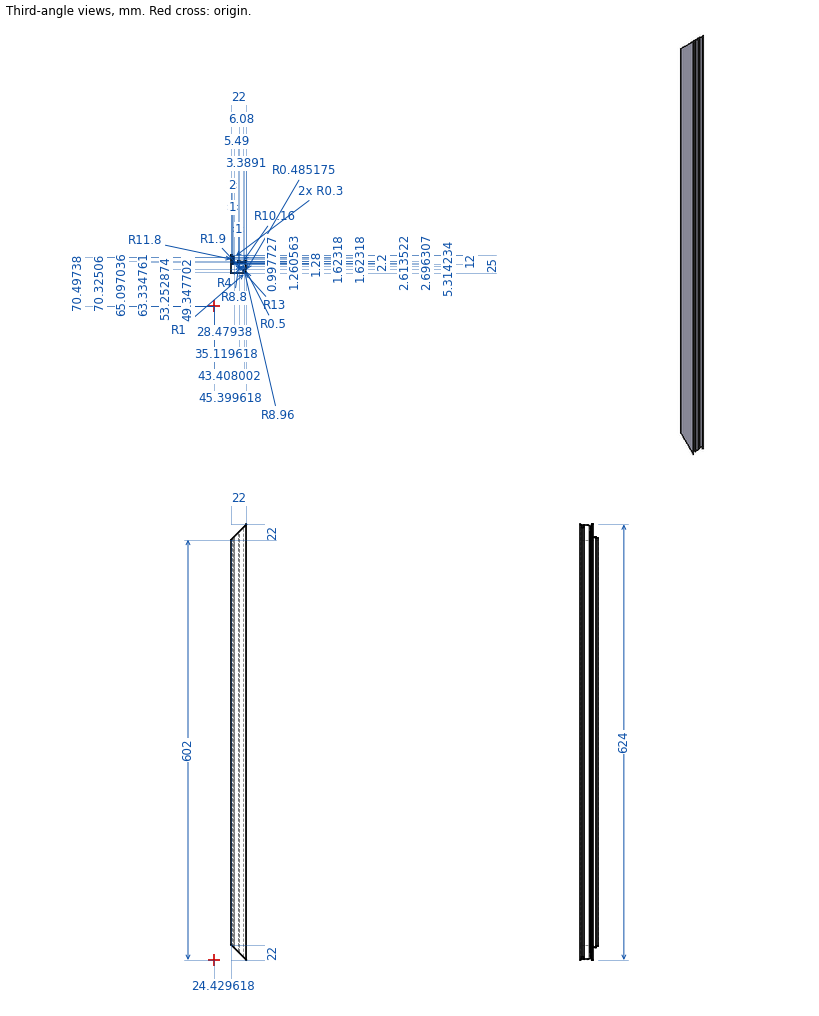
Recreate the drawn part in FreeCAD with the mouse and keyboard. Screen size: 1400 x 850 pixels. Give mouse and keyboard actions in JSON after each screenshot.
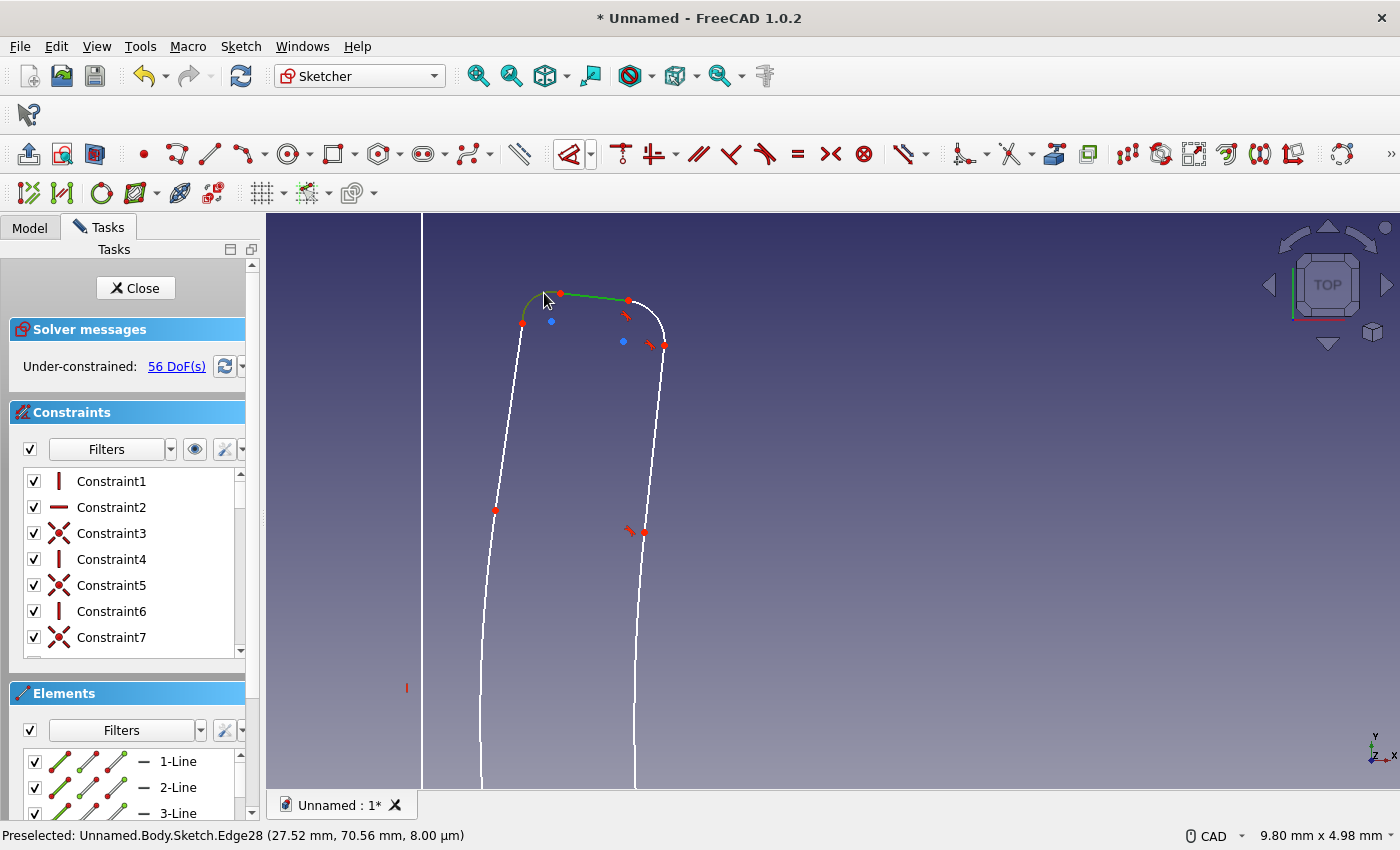
{"action": "key", "text": "t"}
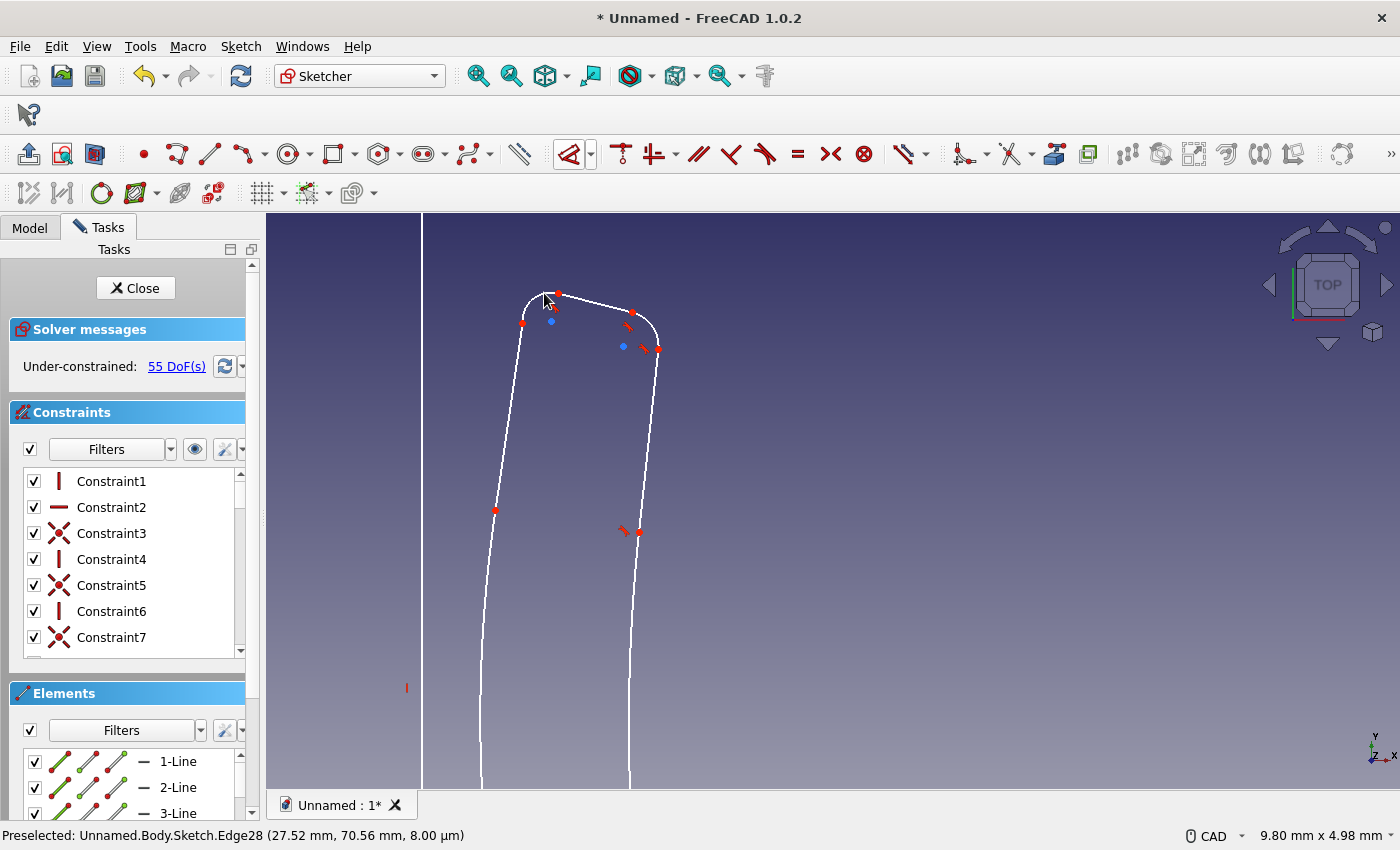
{"action": "scroll", "coordinate": [655, 355], "scroll_direction": "down", "scroll_amount": 10}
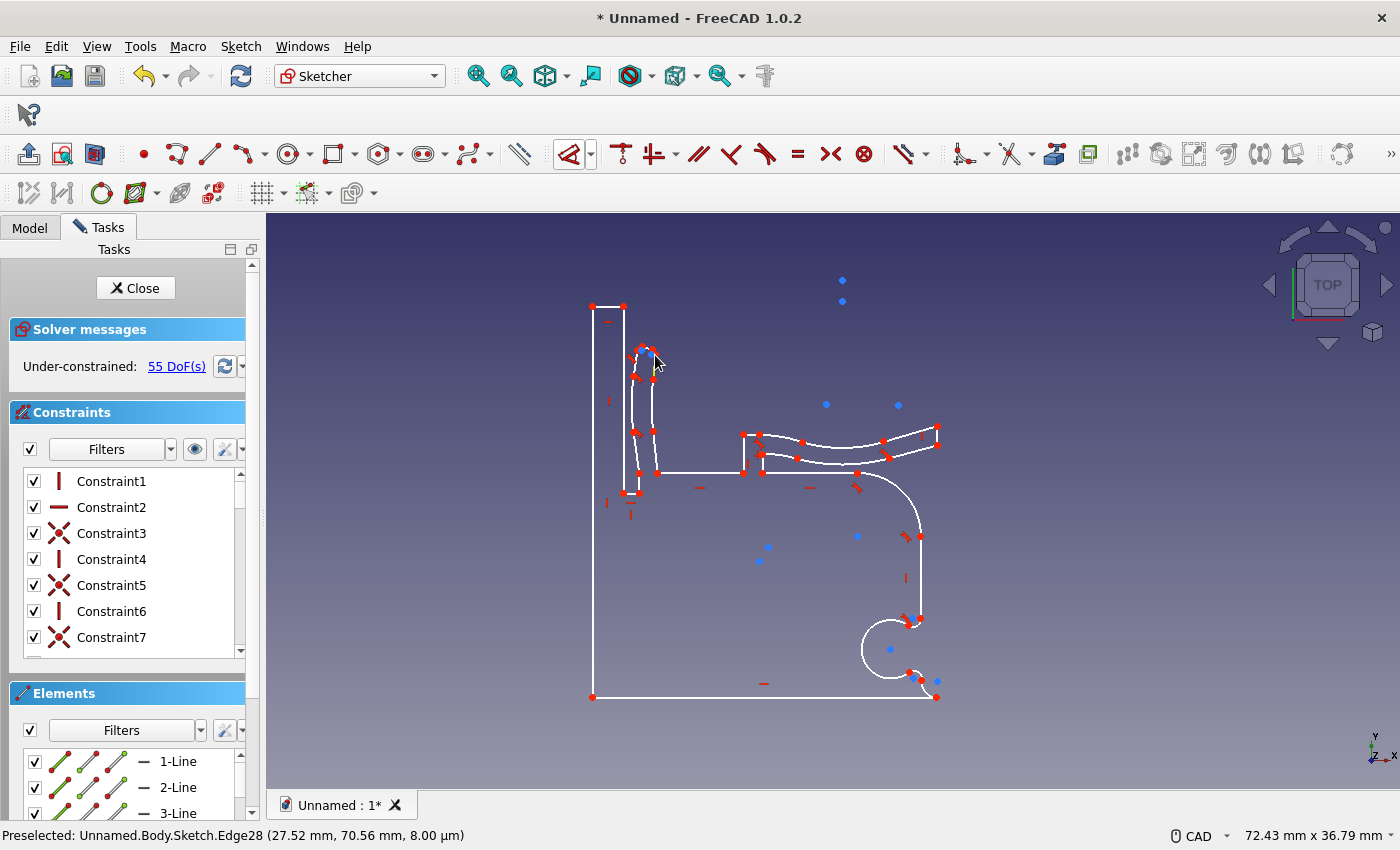
{"action": "scroll", "coordinate": [636, 359], "scroll_direction": "up", "scroll_amount": 3}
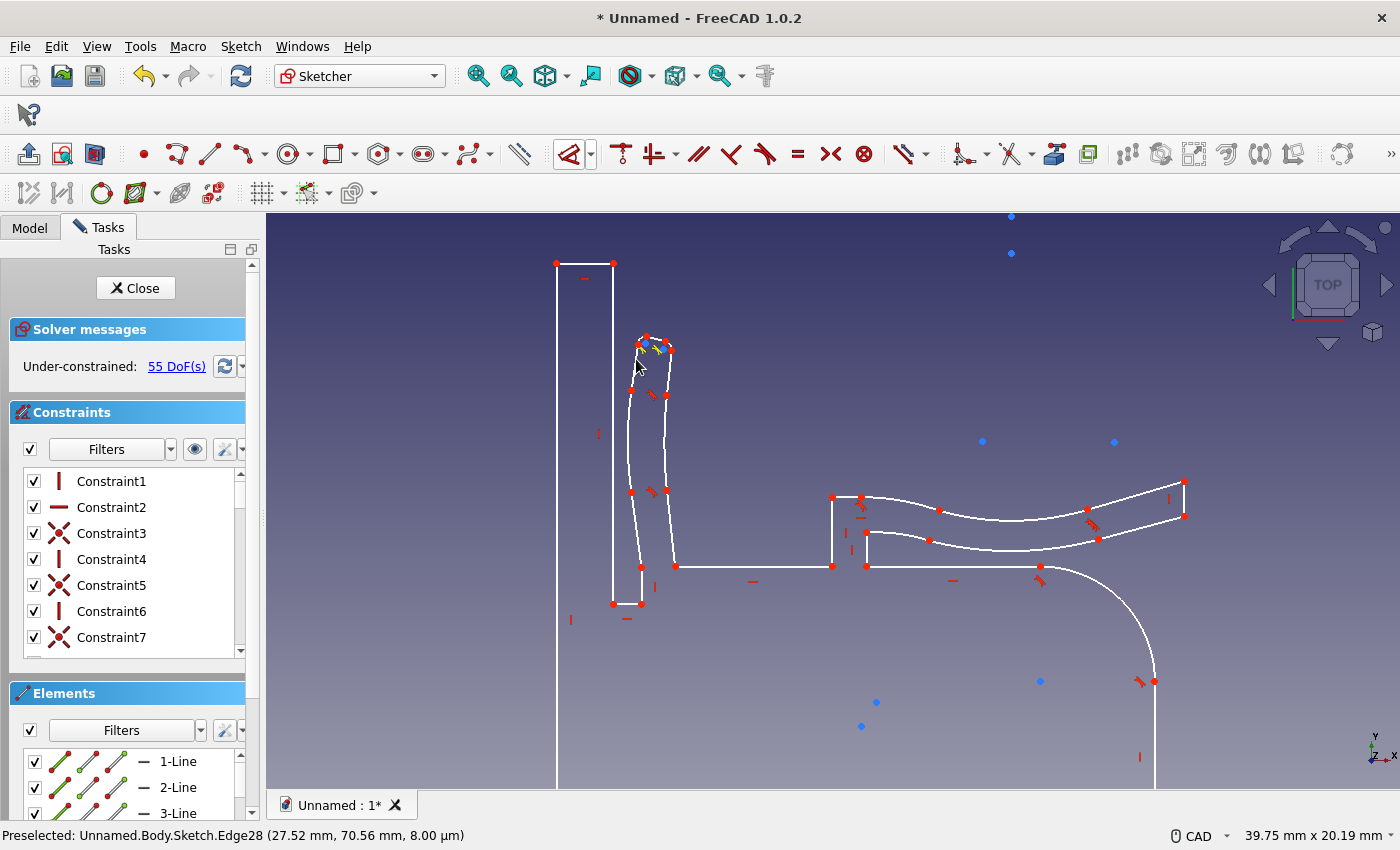
{"action": "left_click", "coordinate": [636, 358]}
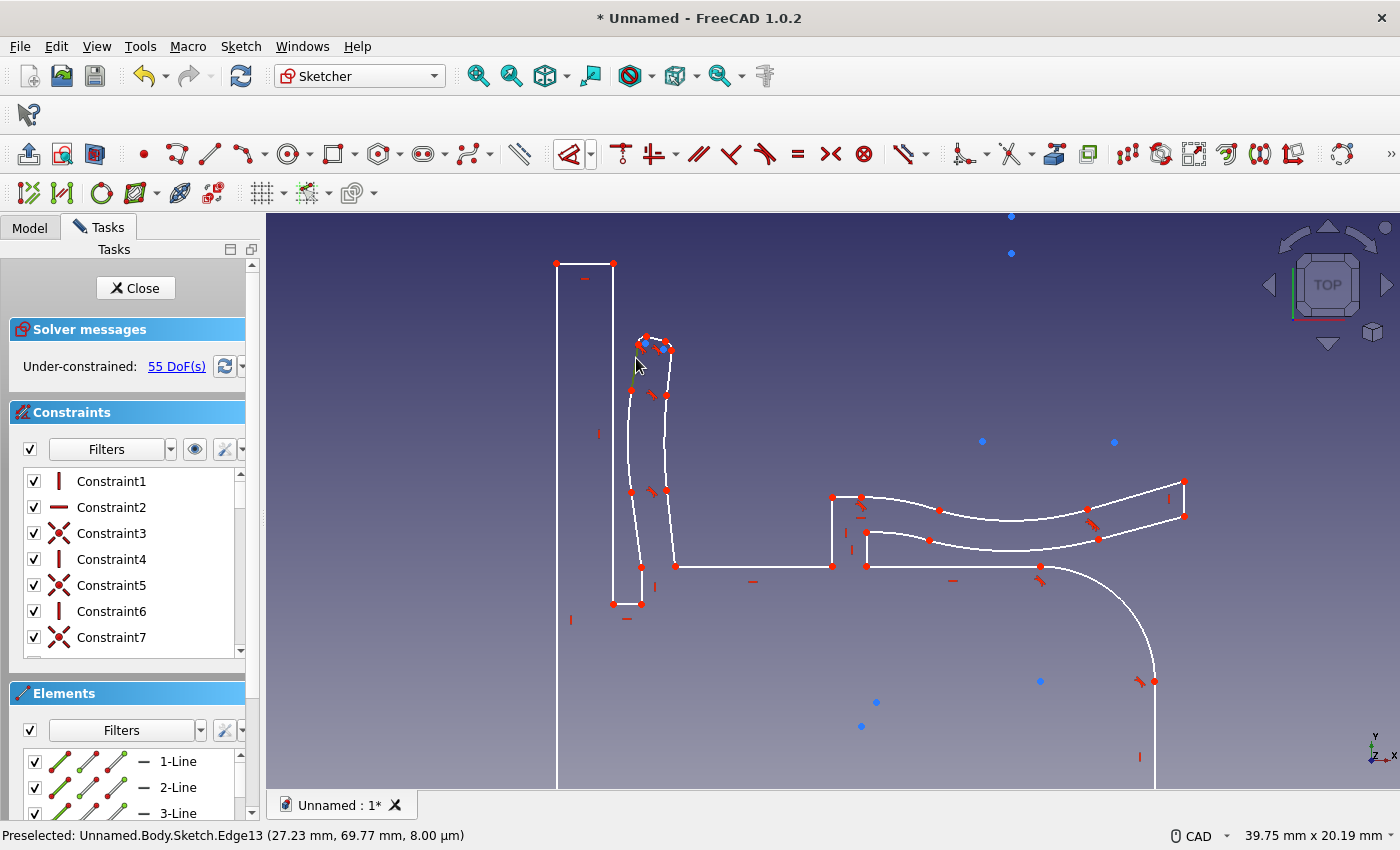
{"action": "scroll", "coordinate": [641, 338], "scroll_direction": "up", "scroll_amount": 4}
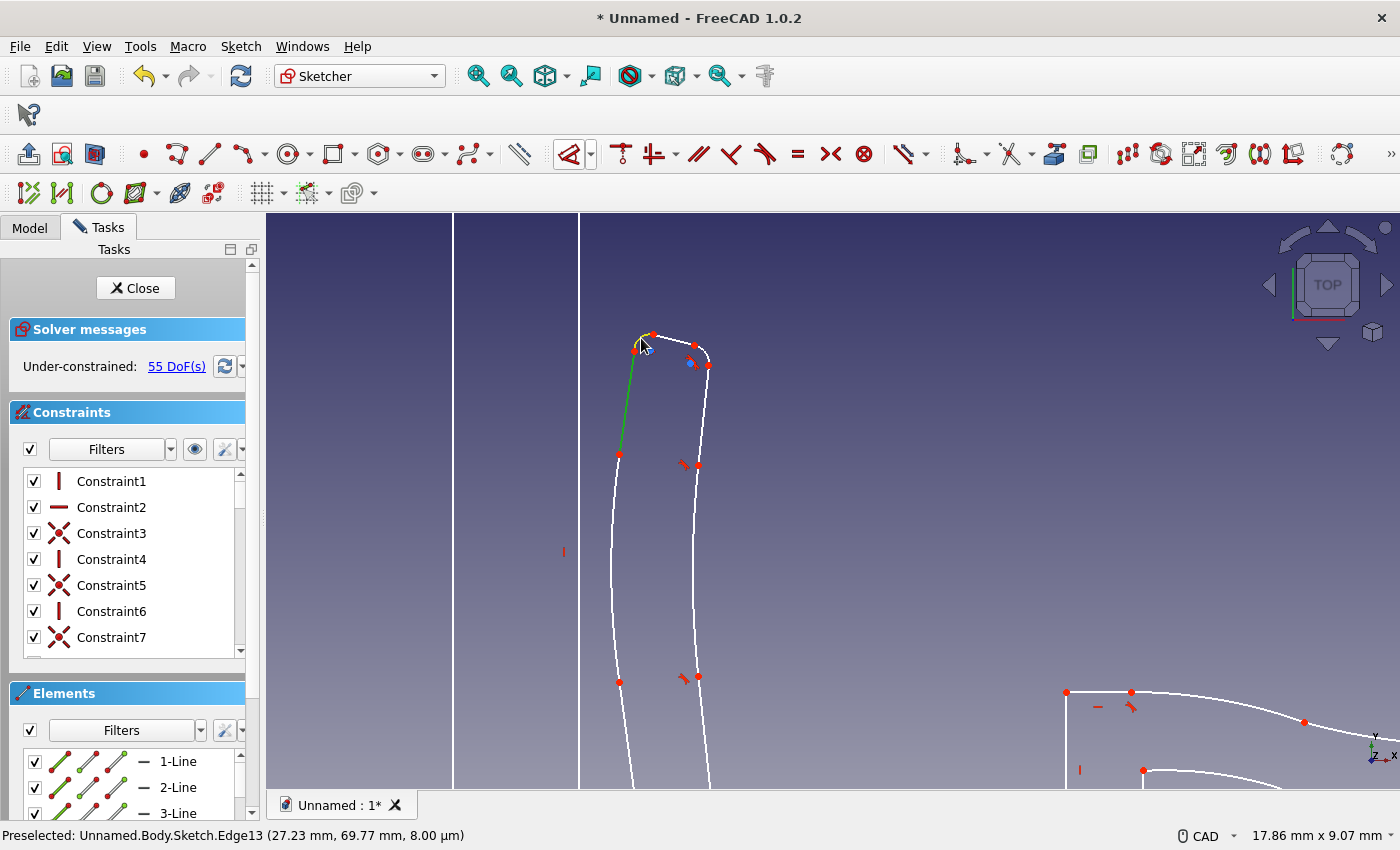
{"action": "left_click", "coordinate": [640, 338]}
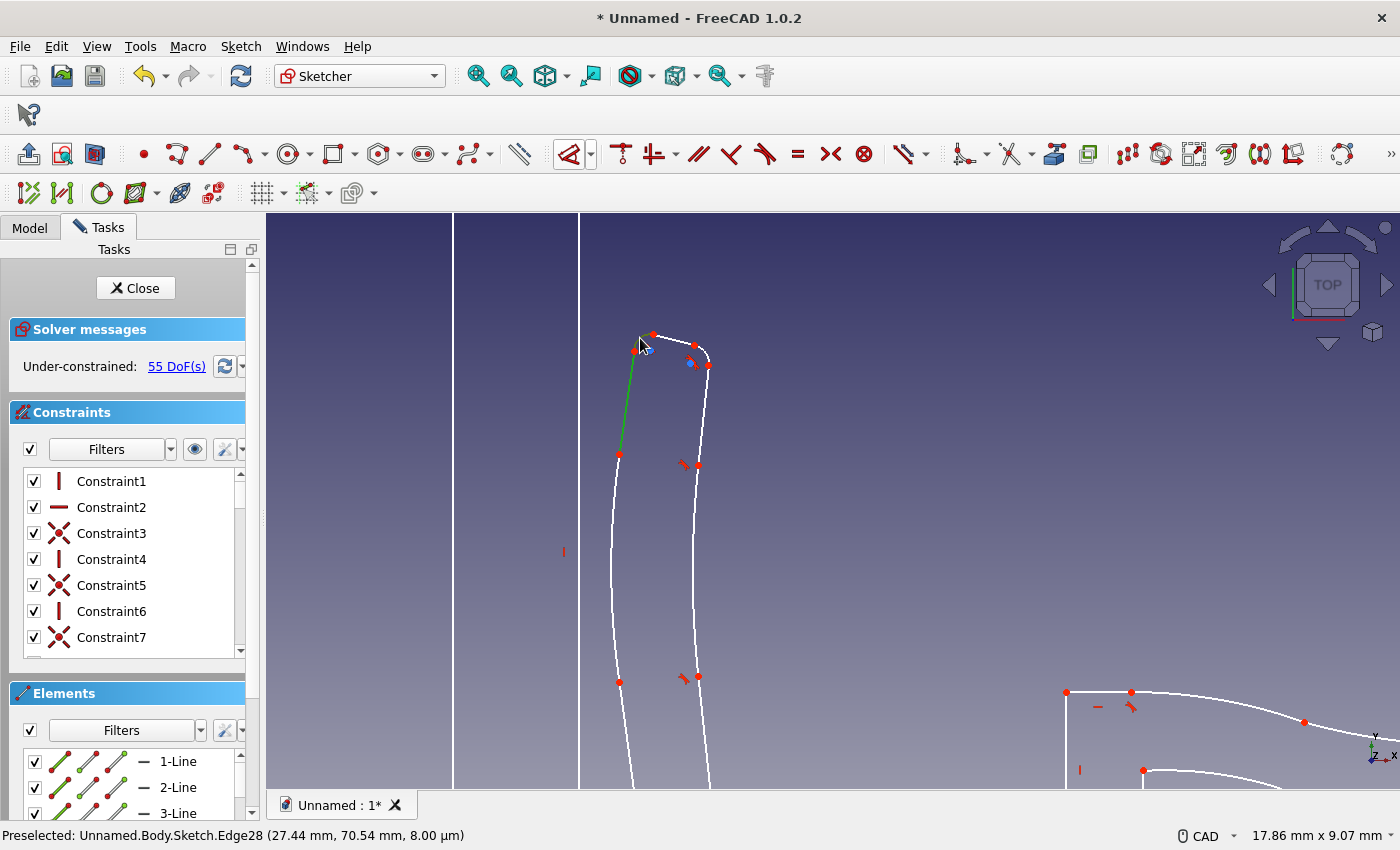
{"action": "left_click", "coordinate": [765, 154]}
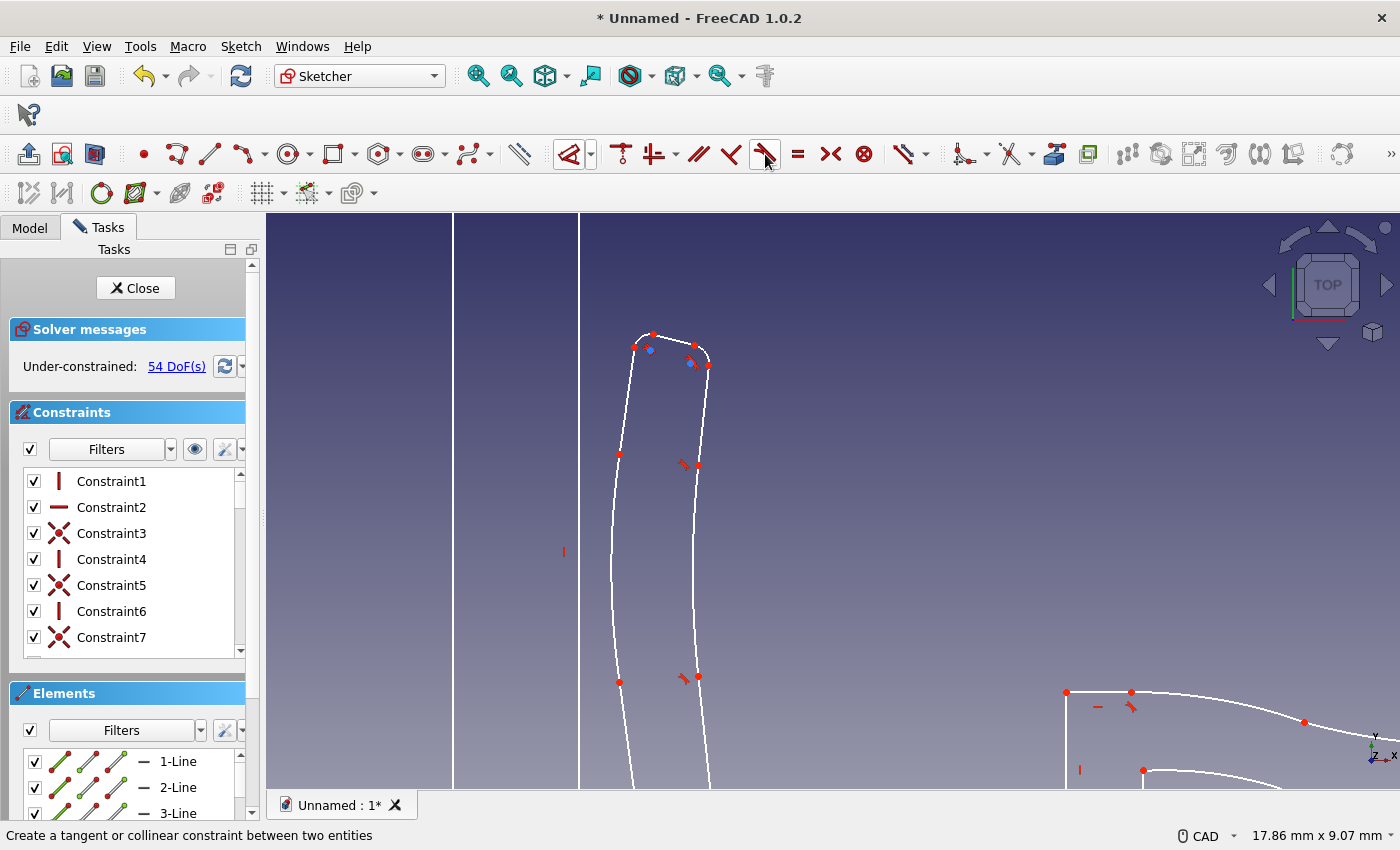
{"action": "left_click", "coordinate": [630, 380]}